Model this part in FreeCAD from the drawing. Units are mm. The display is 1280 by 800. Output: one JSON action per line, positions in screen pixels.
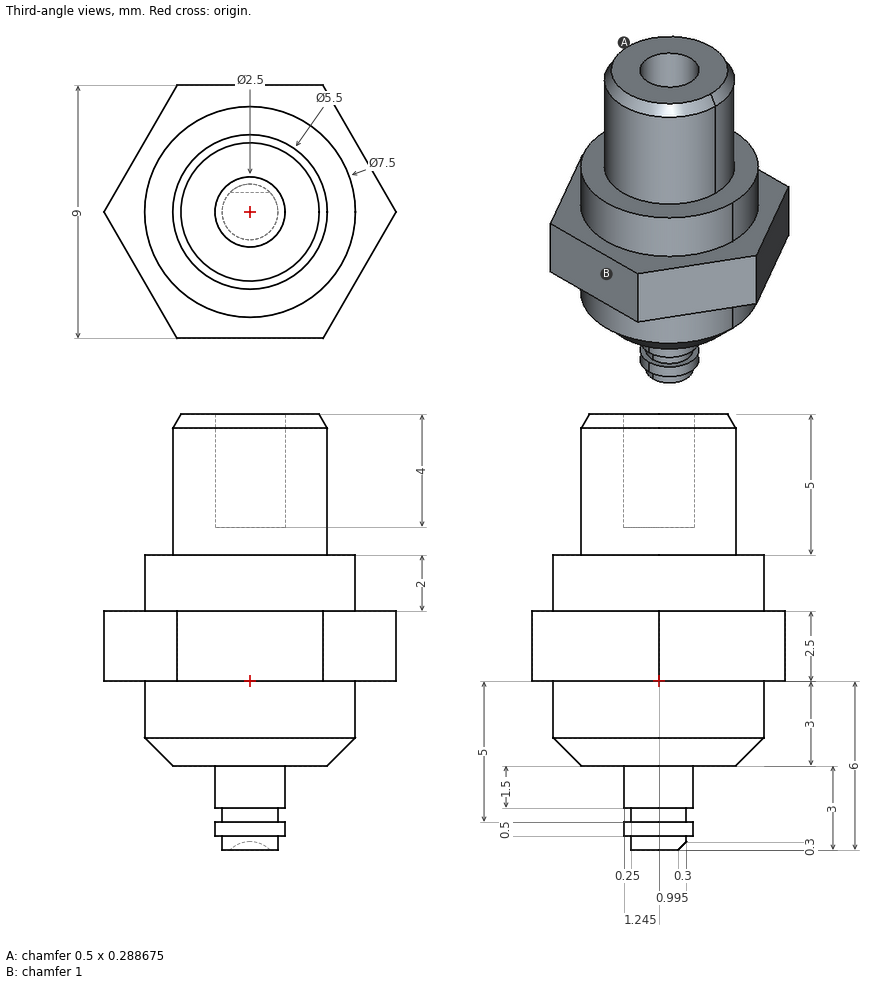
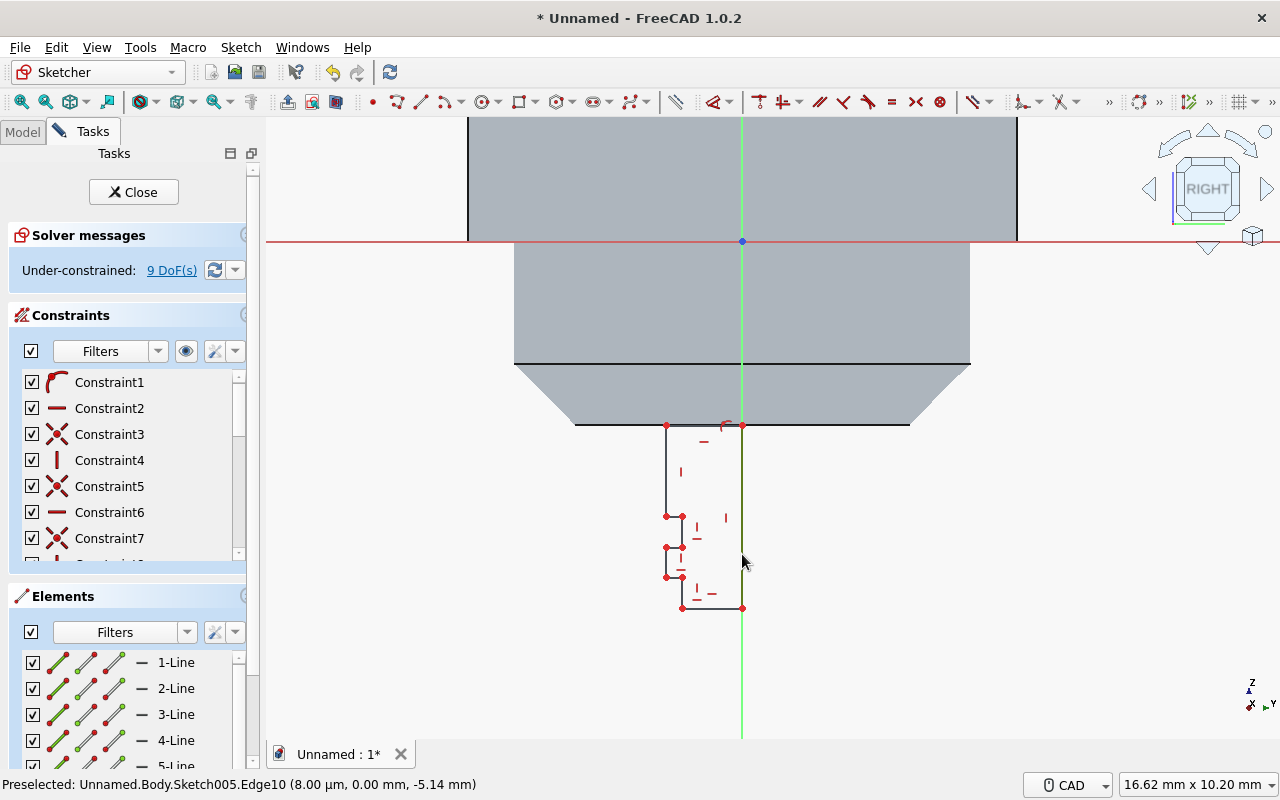
{"action": "key", "text": "i"}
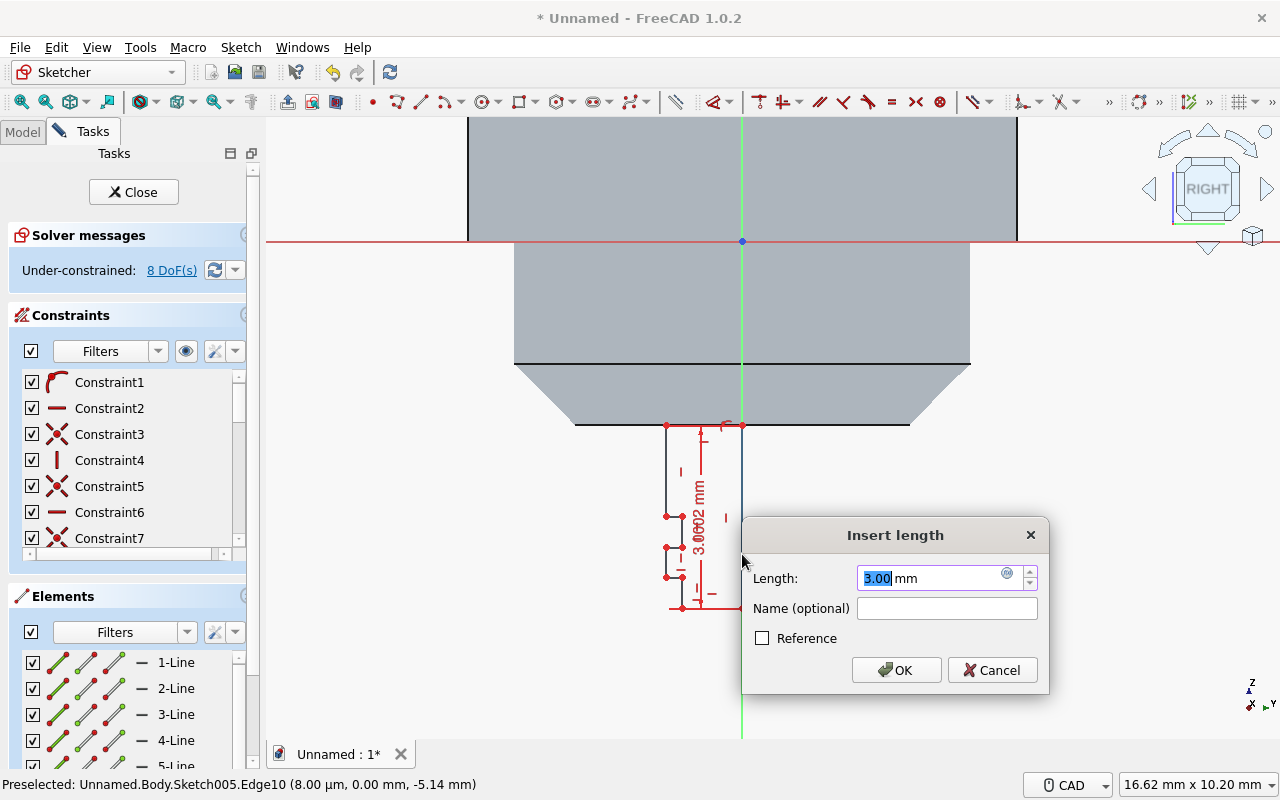
{"action": "type", "text": "3"}
{"action": "key", "text": "Return"}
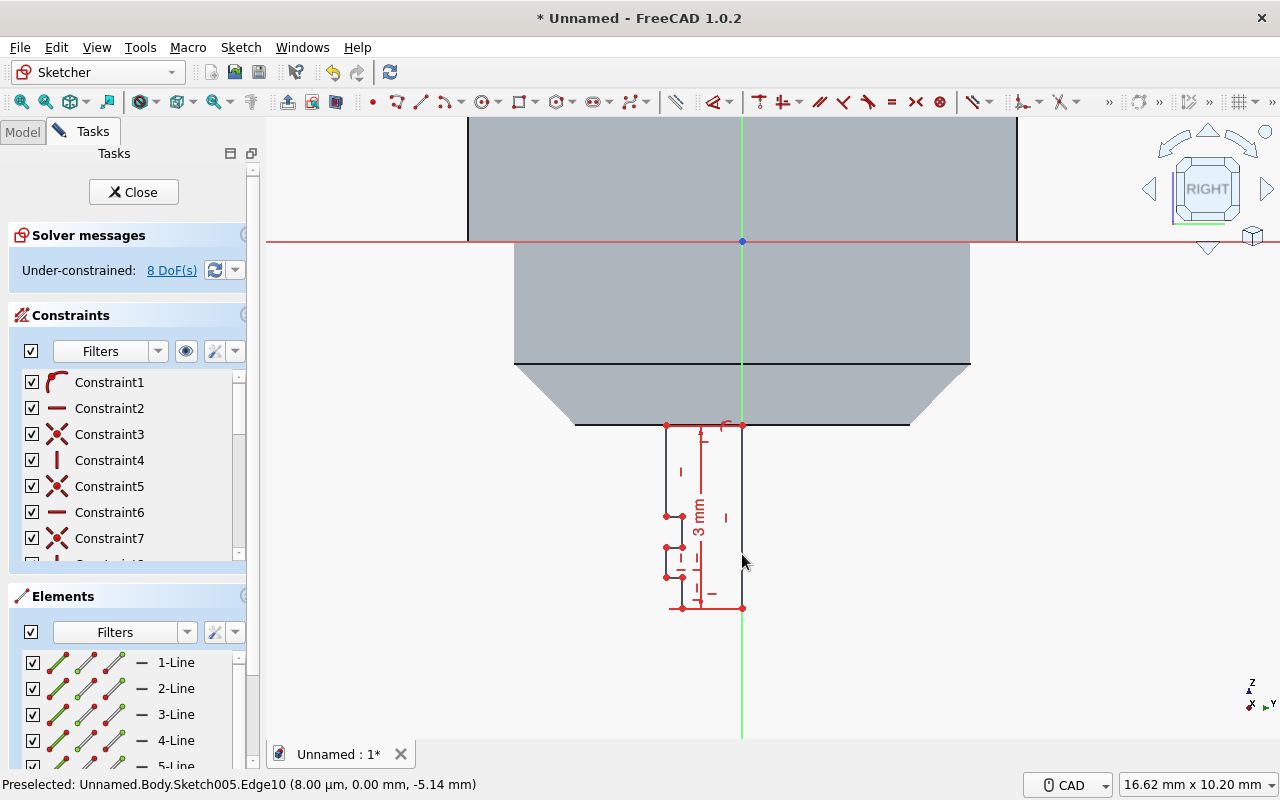
{"action": "left_click", "coordinate": [742, 426]}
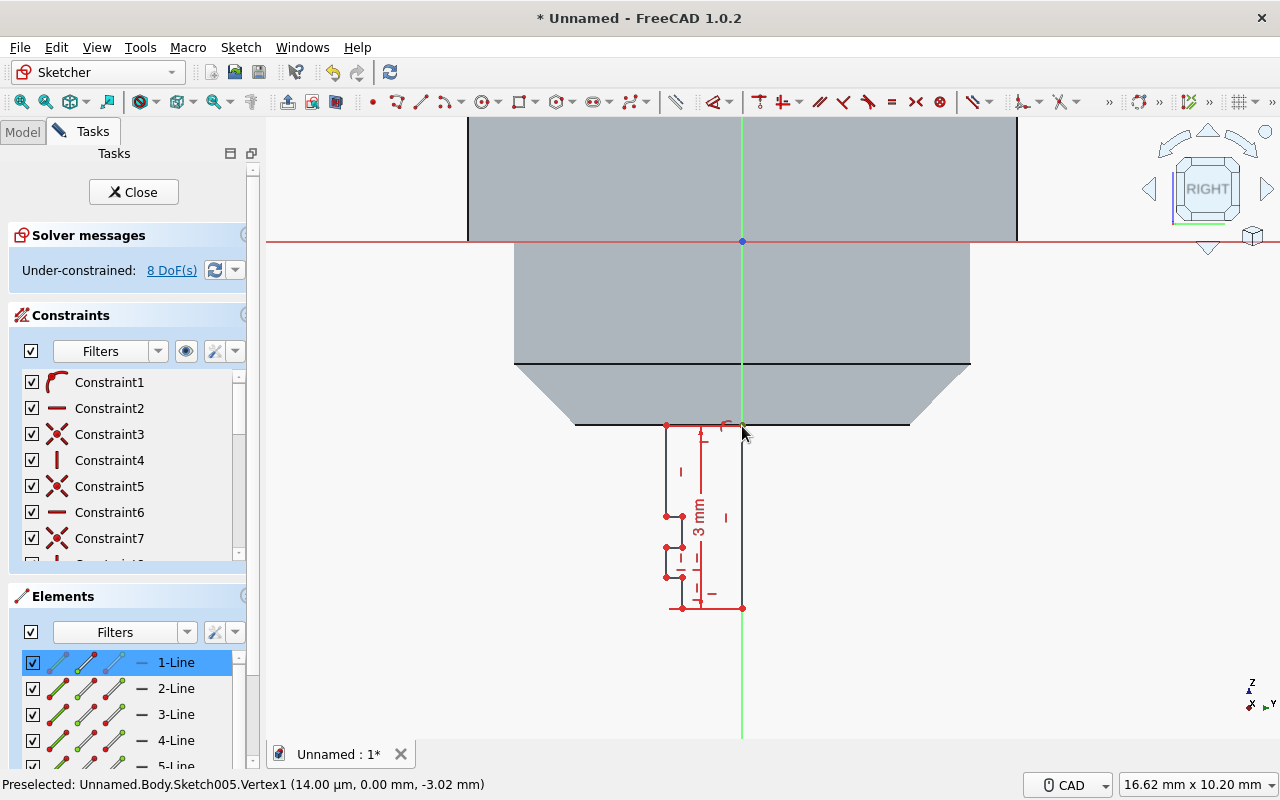
{"action": "key", "text": "i"}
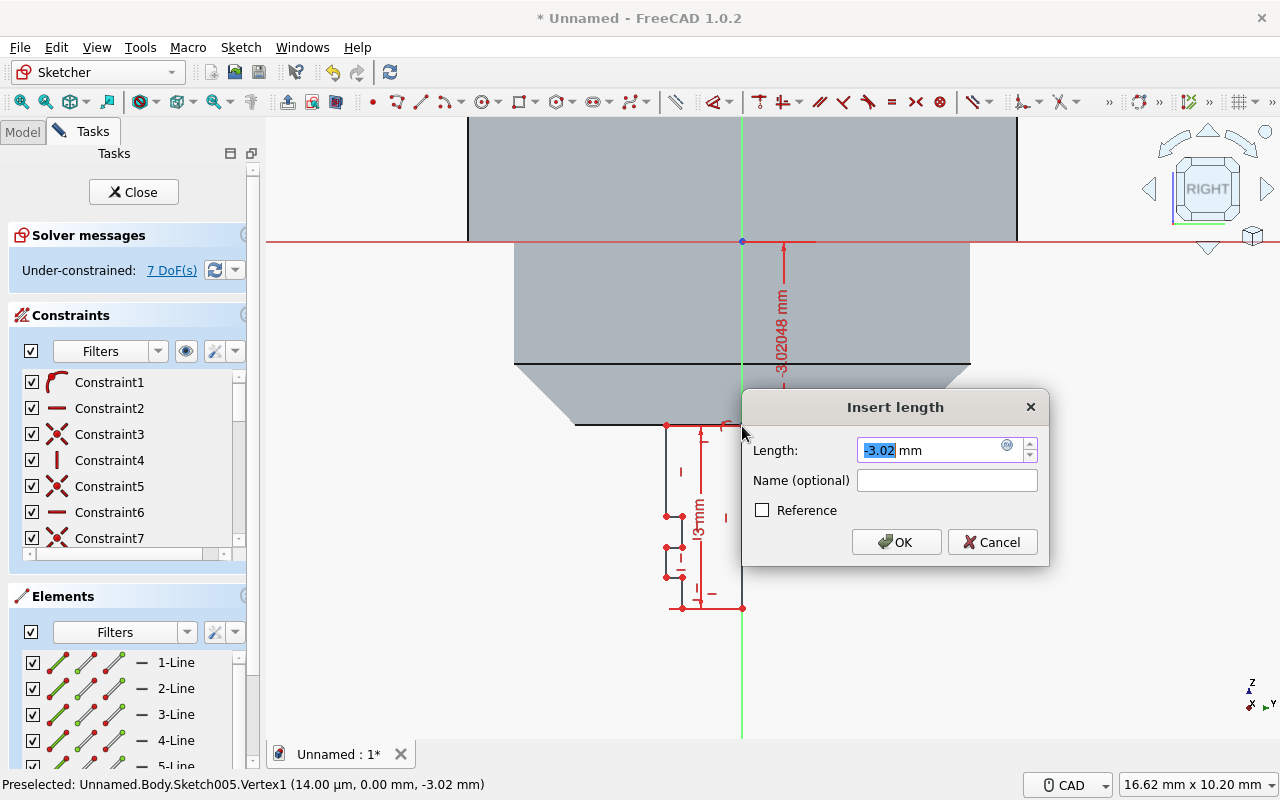
{"action": "type", "text": "-3"}
{"action": "key", "text": "Return"}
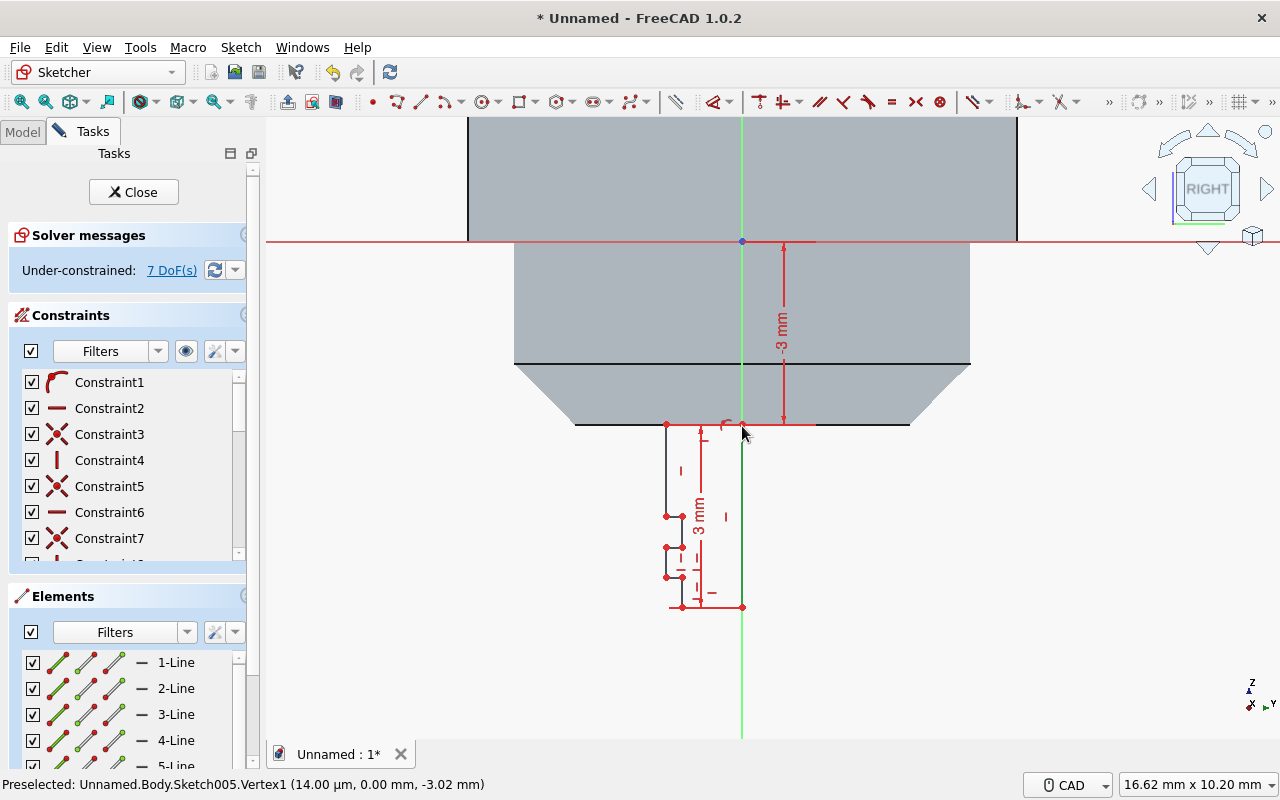
{"action": "left_click", "coordinate": [682, 548]}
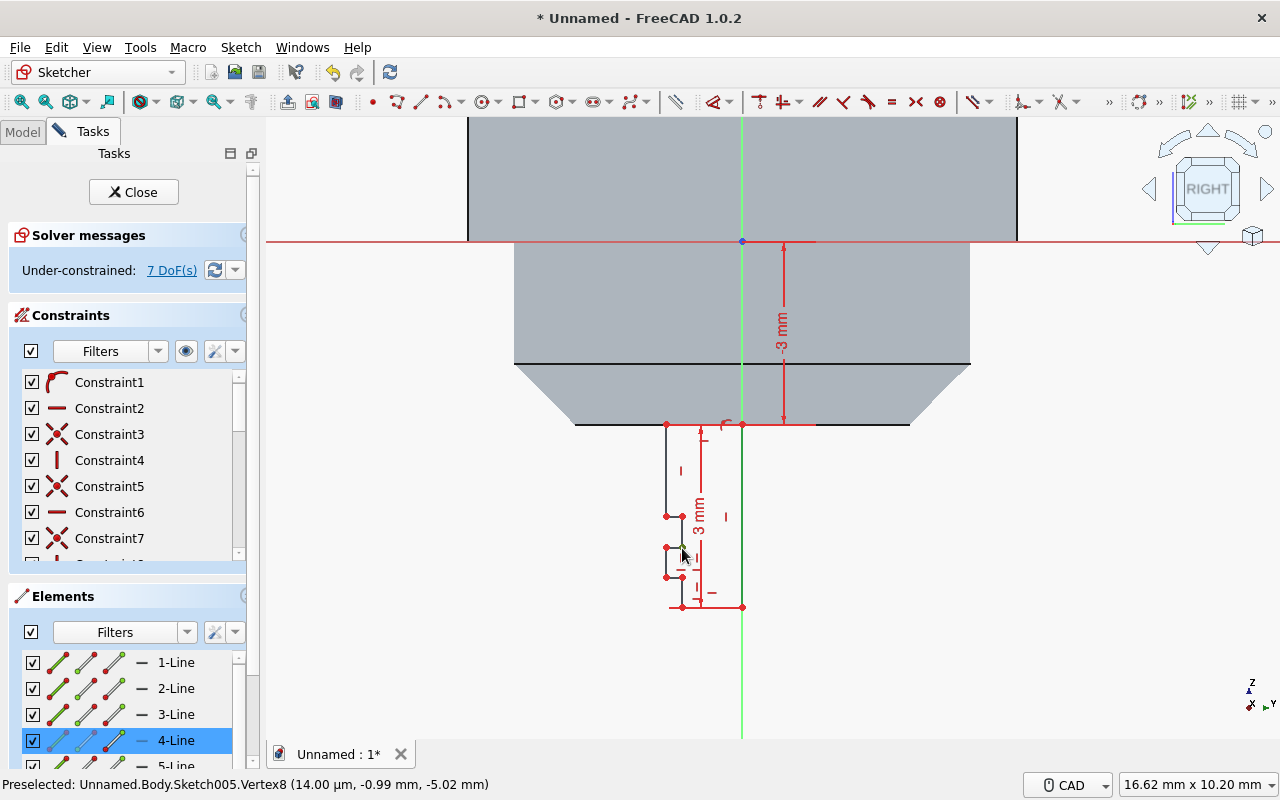
{"action": "key", "text": "i"}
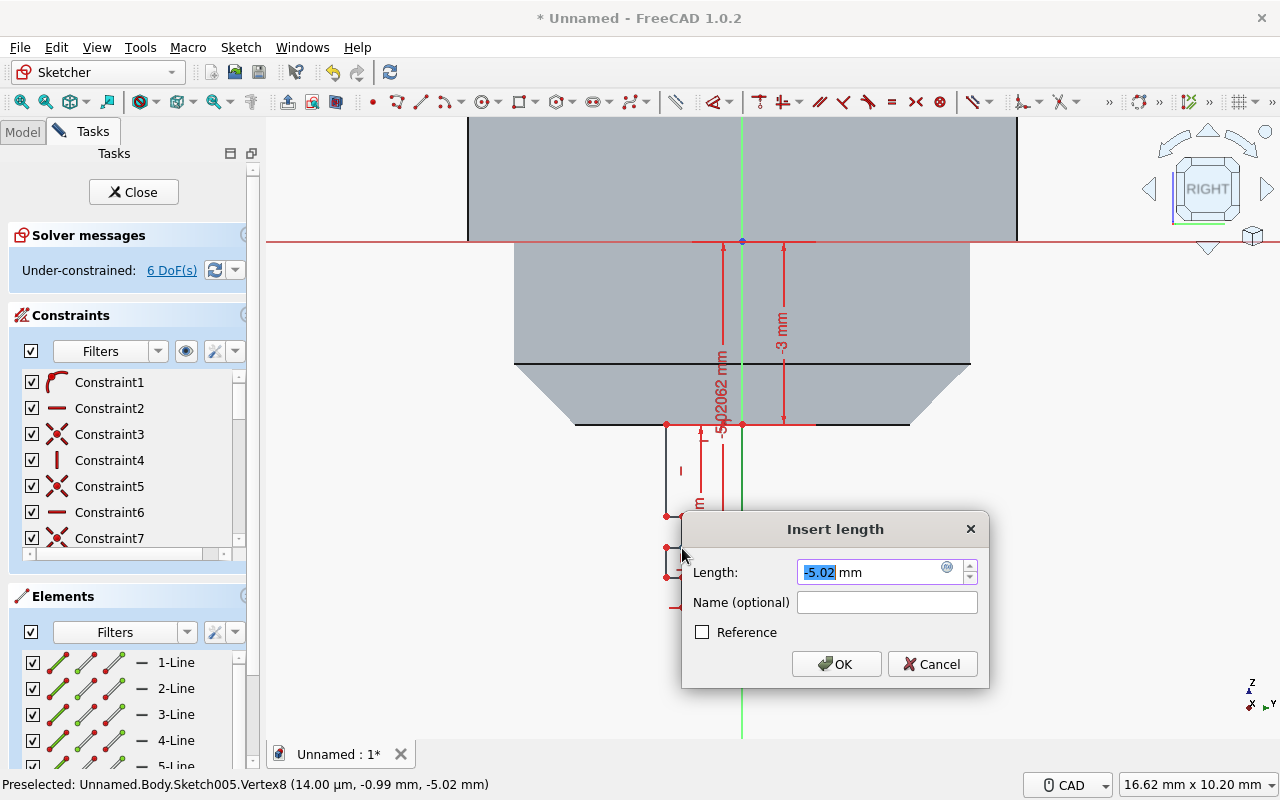
{"action": "type", "text": "-5"}
{"action": "key", "text": "Return"}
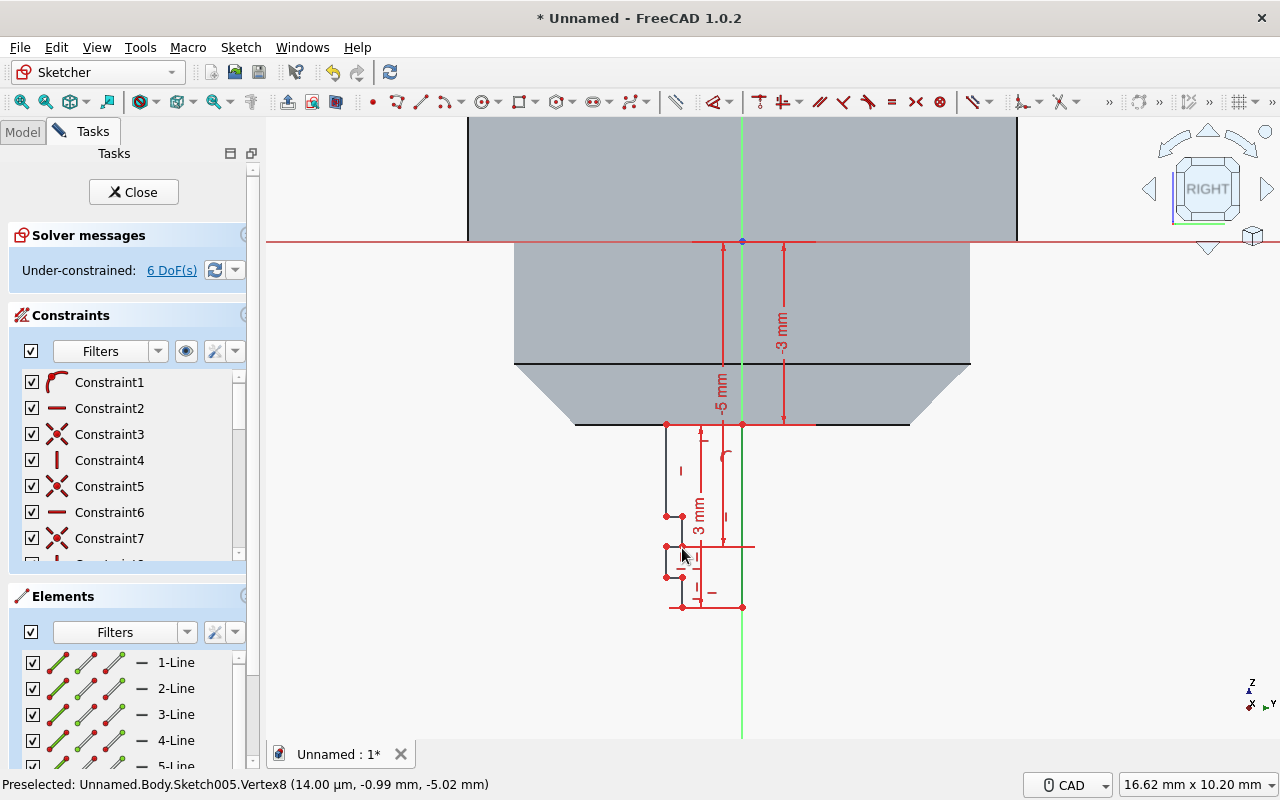
{"action": "left_click", "coordinate": [666, 452]}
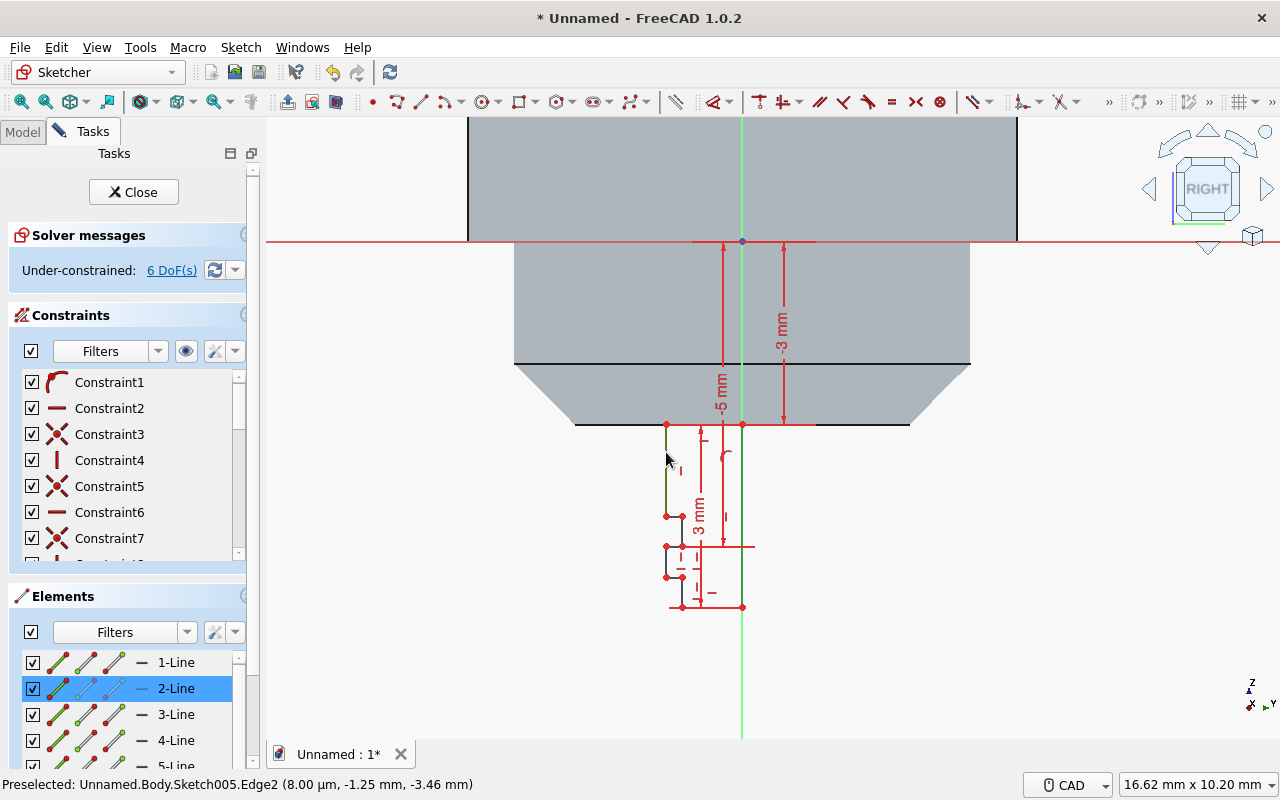
{"action": "left_click", "coordinate": [732, 102]}